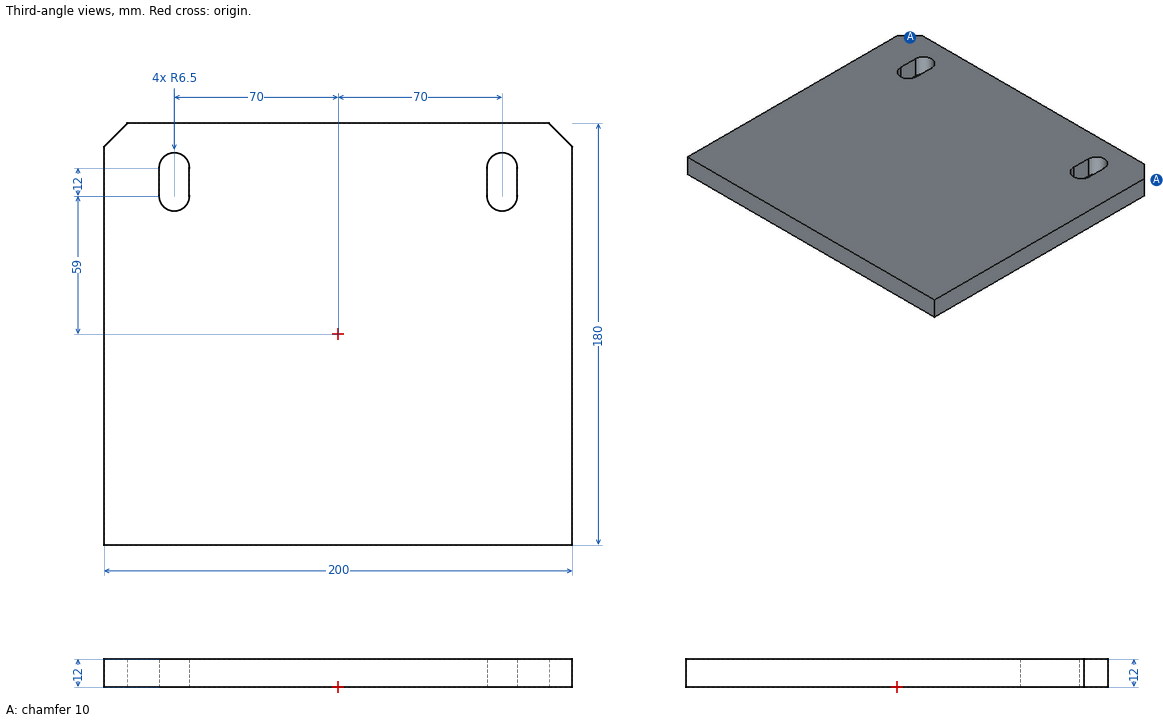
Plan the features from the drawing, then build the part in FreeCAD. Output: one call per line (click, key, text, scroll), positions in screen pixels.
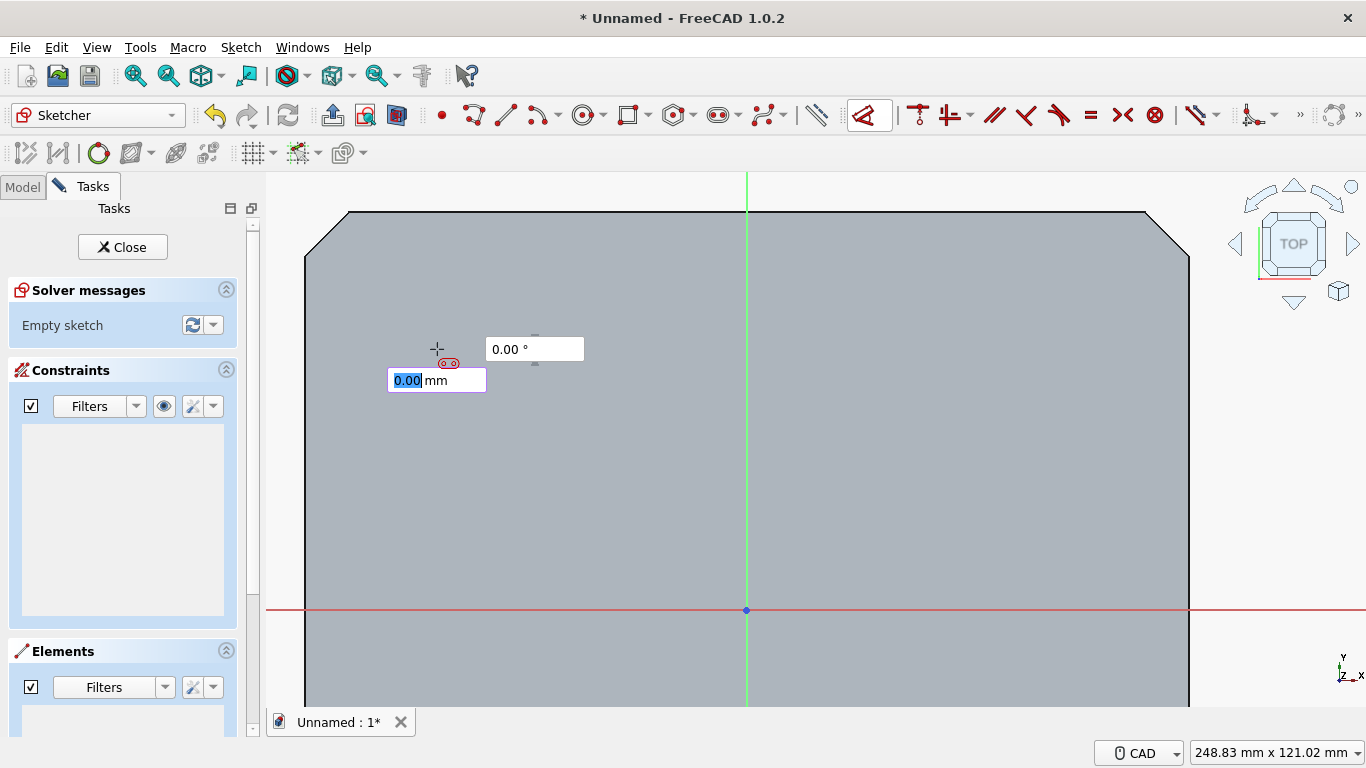
click(437, 296)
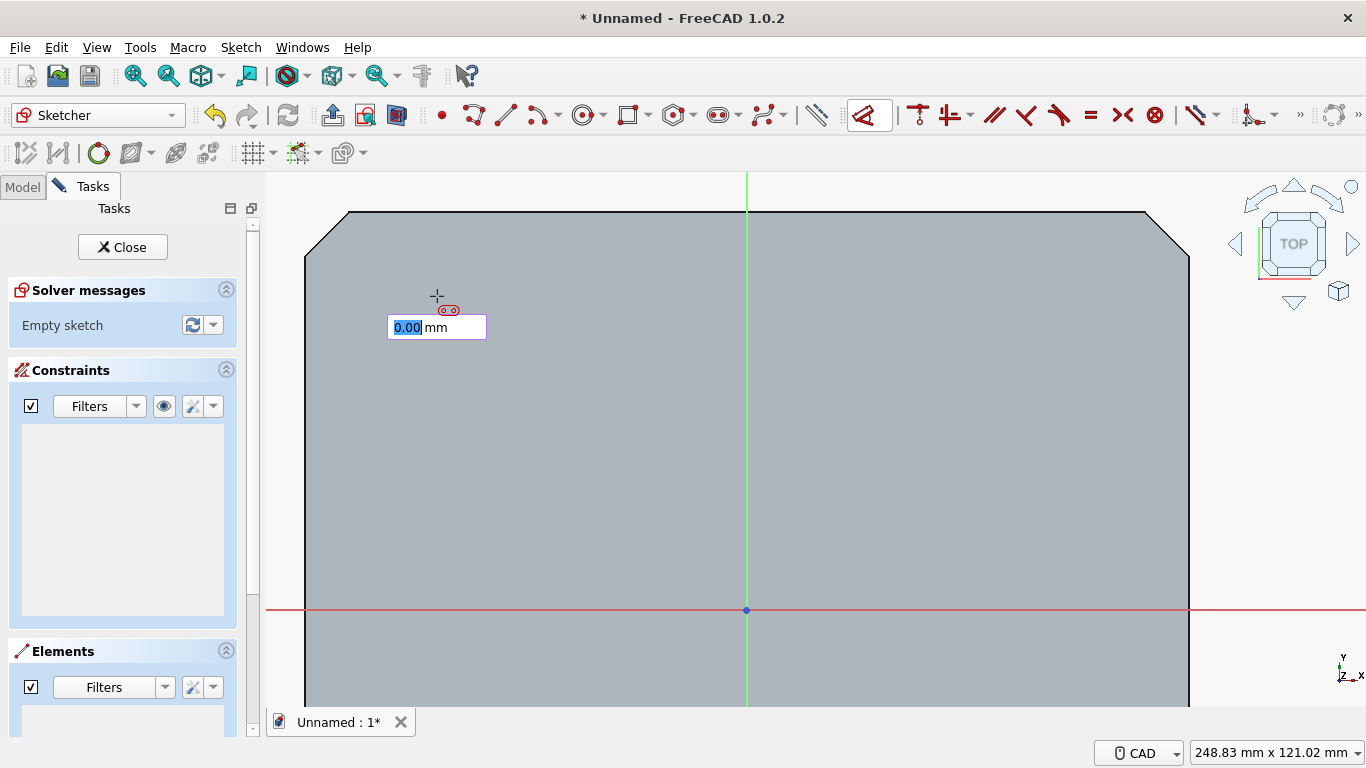
click(466, 323)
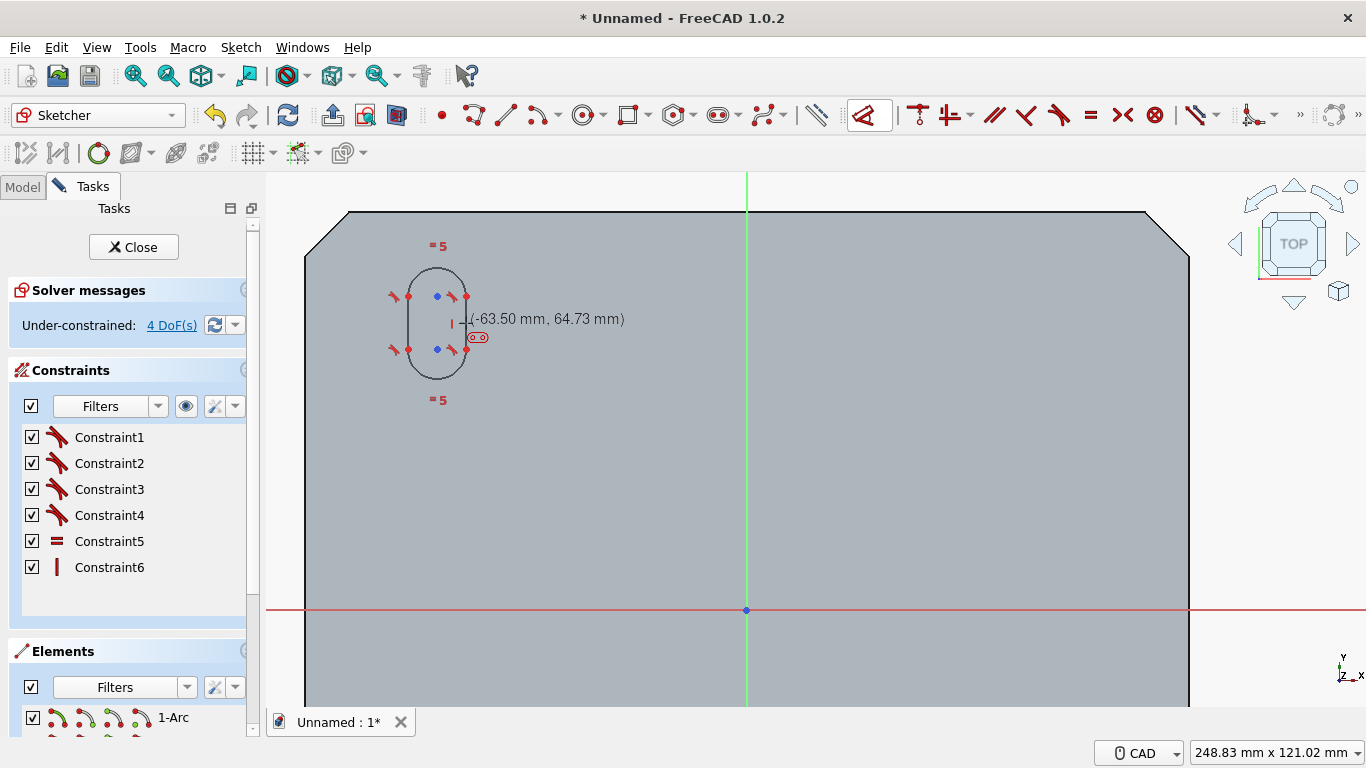
click(1056, 349)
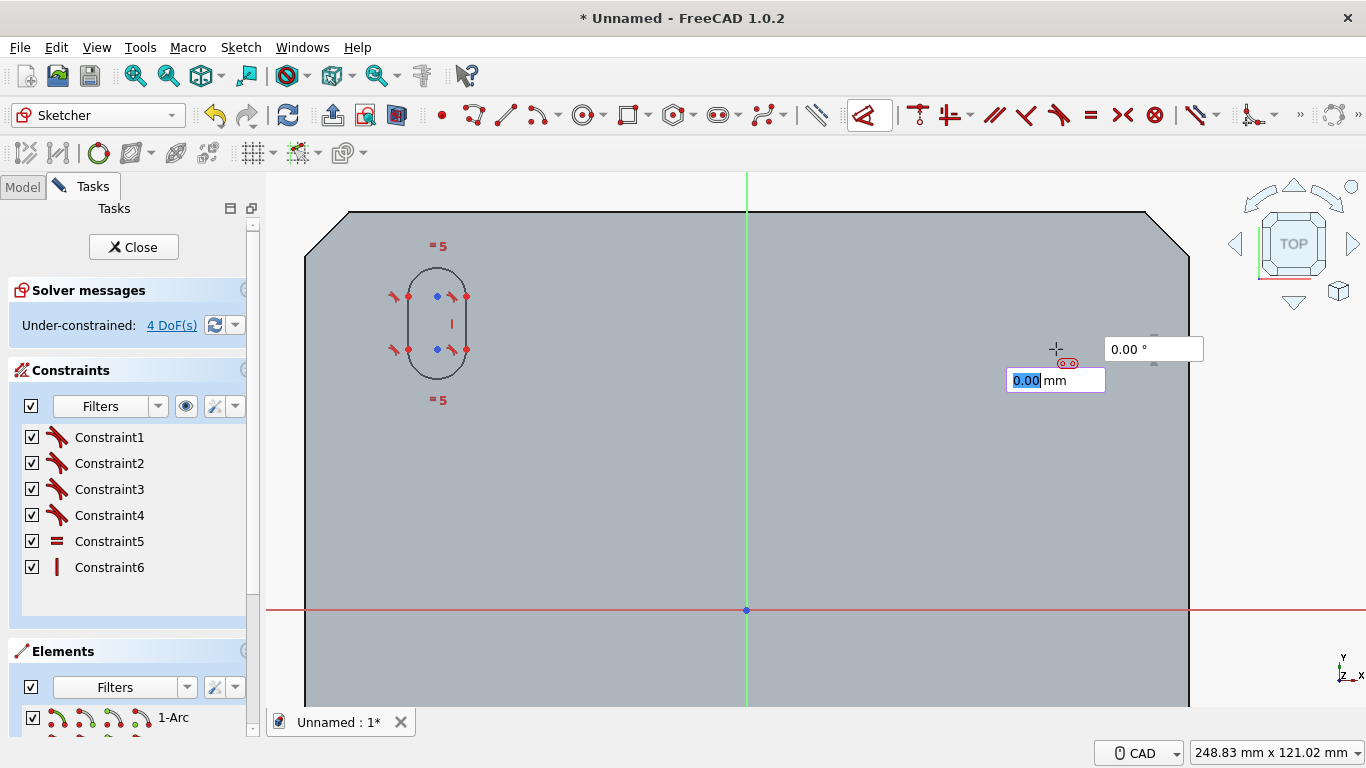
click(1056, 296)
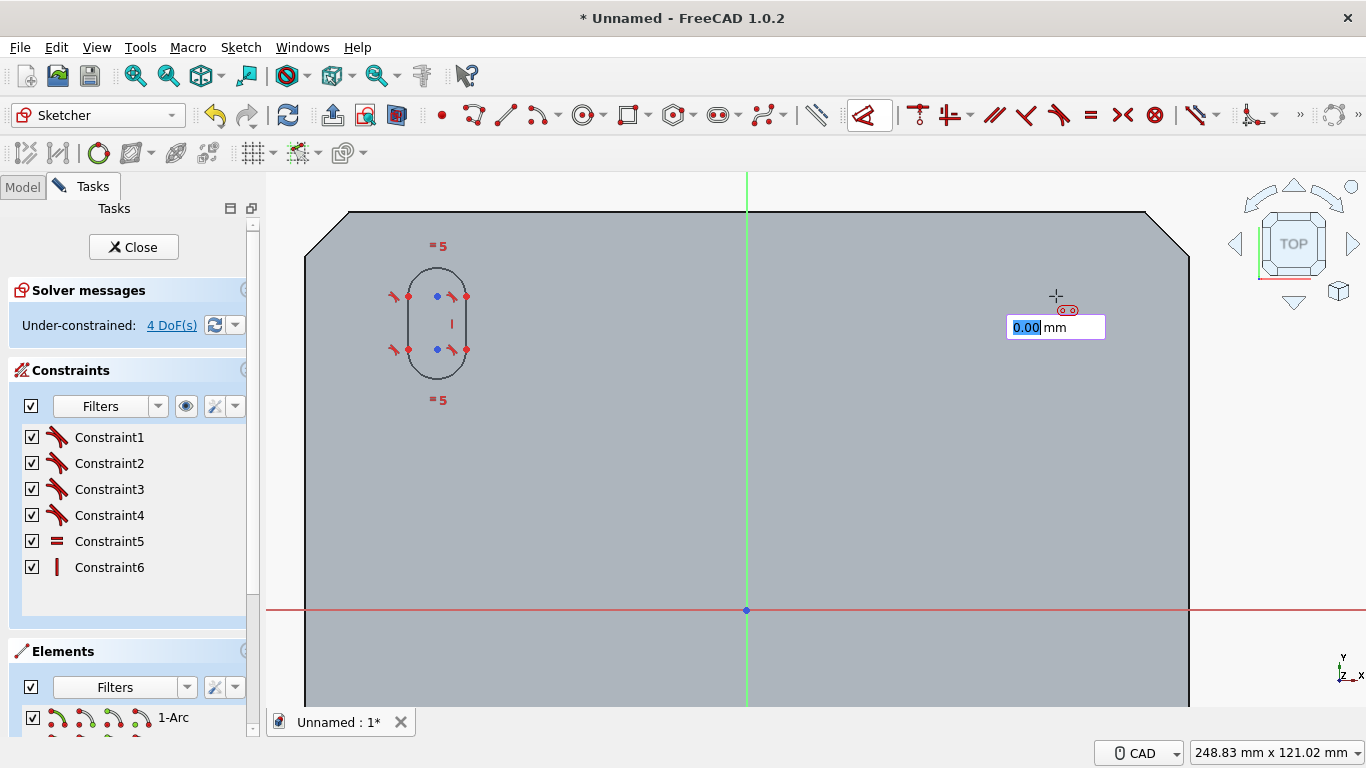
click(1085, 323)
key(Escape)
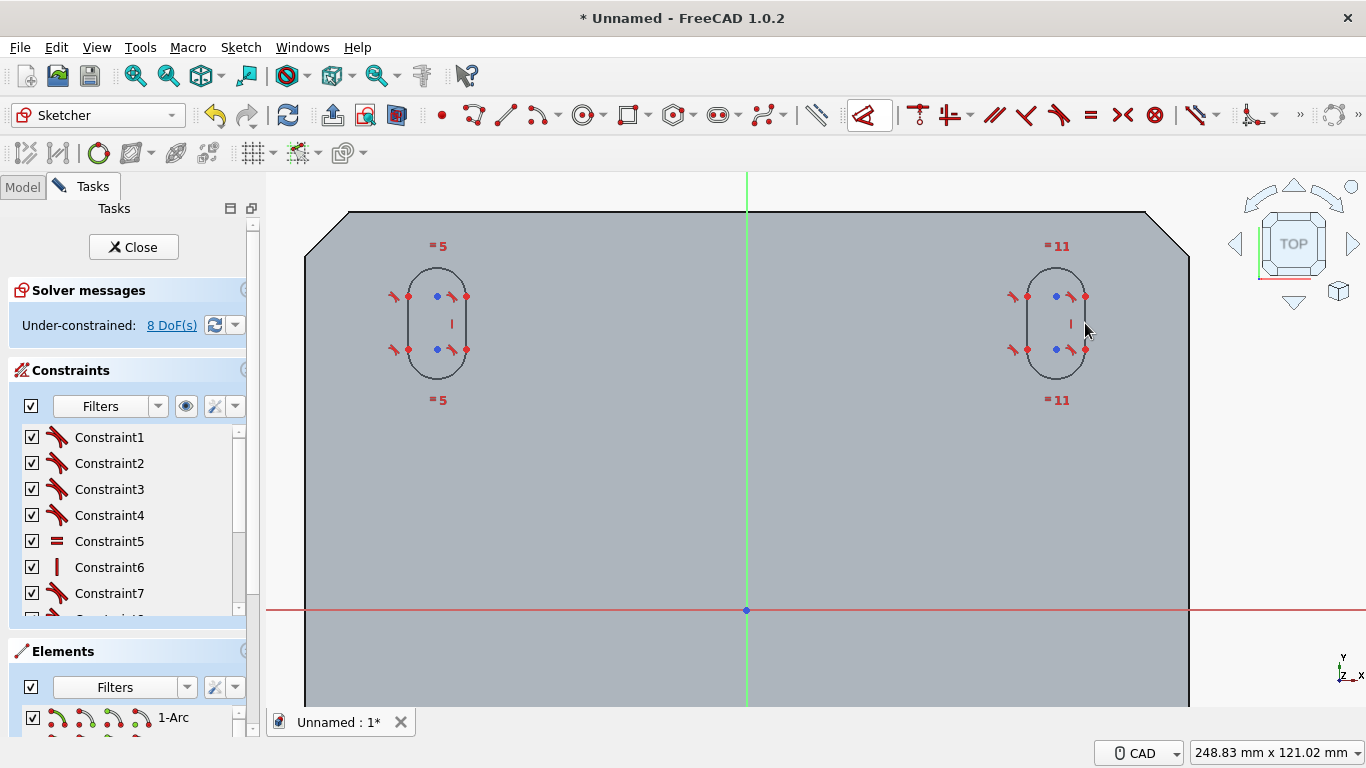
click(420, 373)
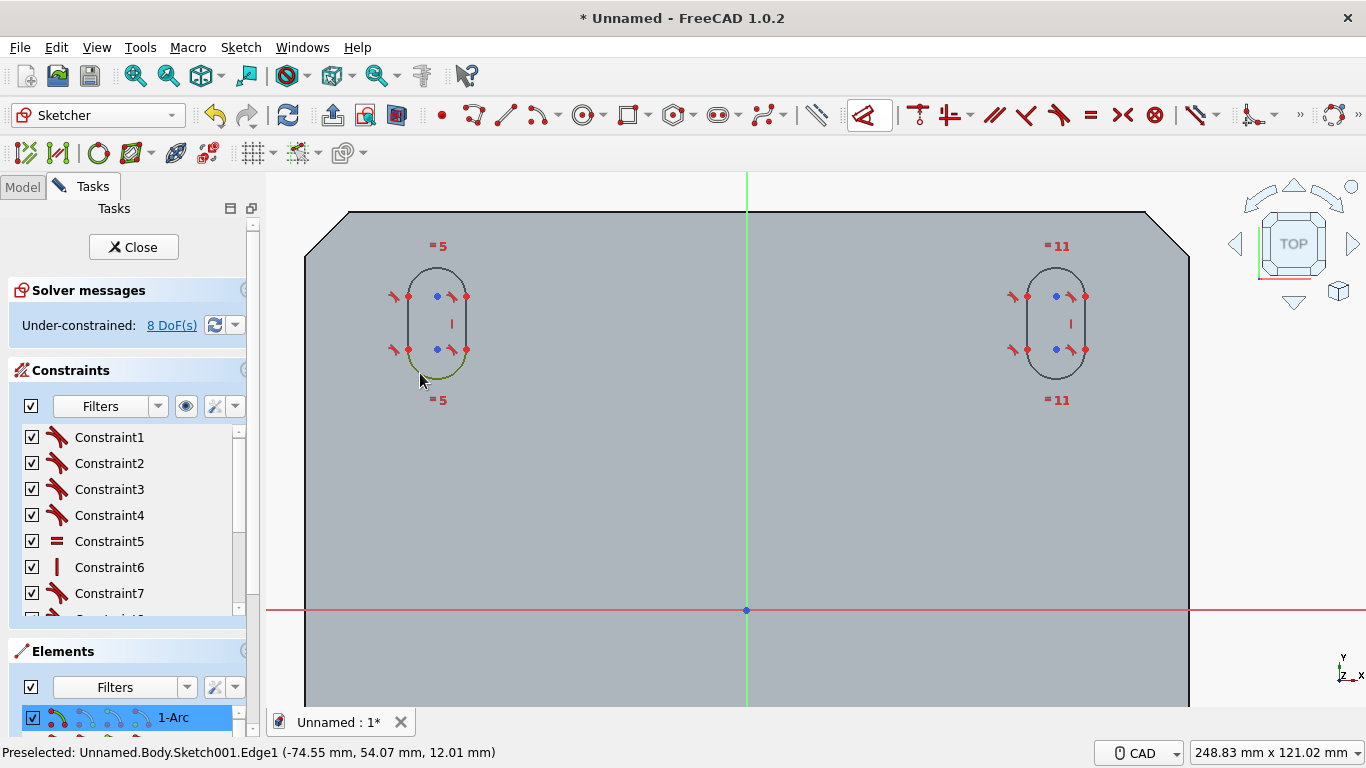
click(1039, 373)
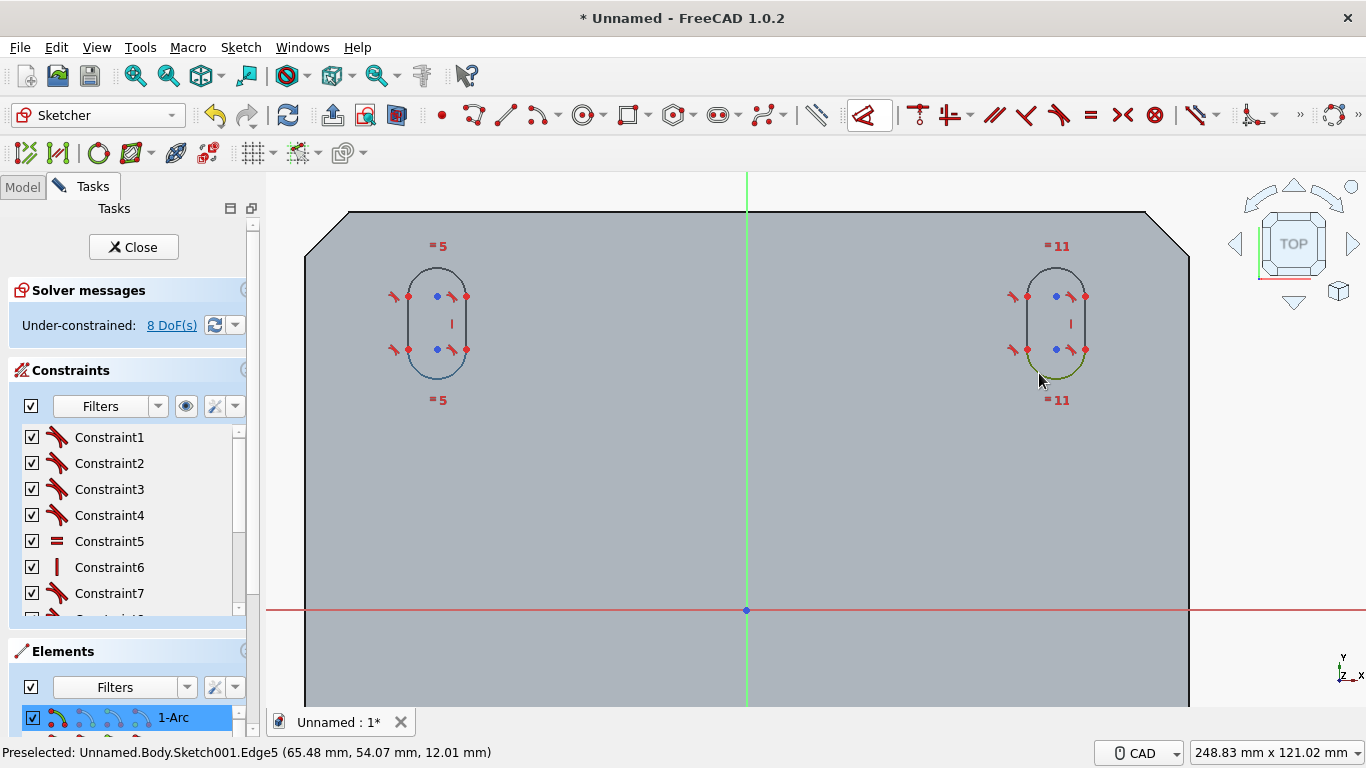
key(e)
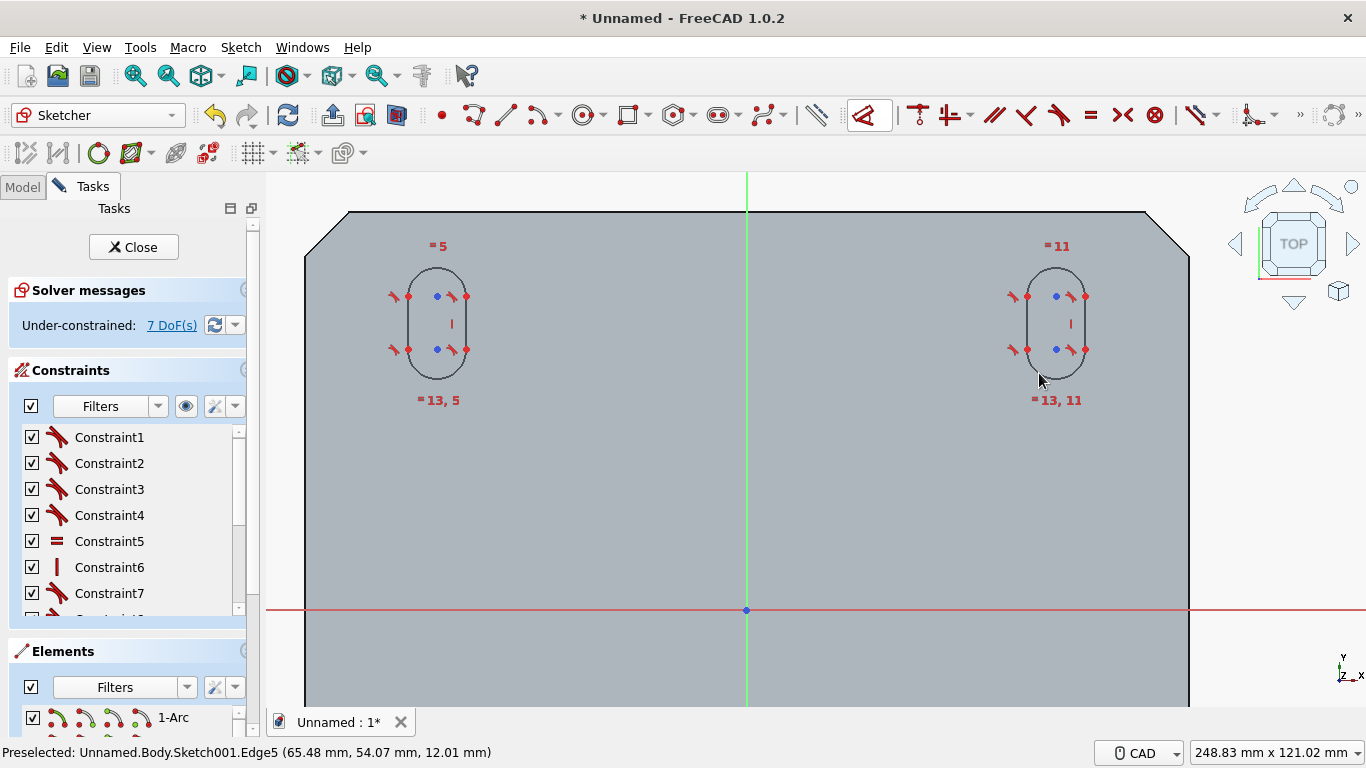
scroll(420, 373, up, 2)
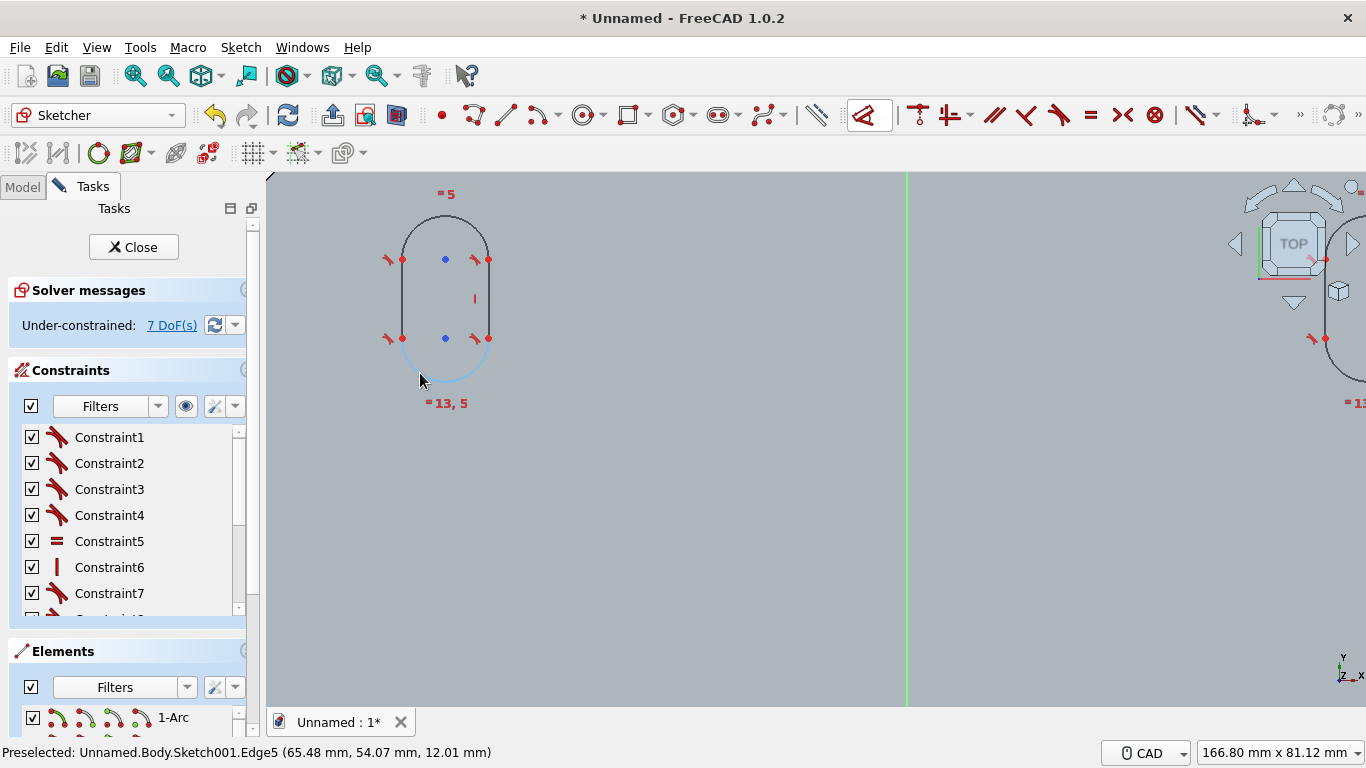
click(420, 374)